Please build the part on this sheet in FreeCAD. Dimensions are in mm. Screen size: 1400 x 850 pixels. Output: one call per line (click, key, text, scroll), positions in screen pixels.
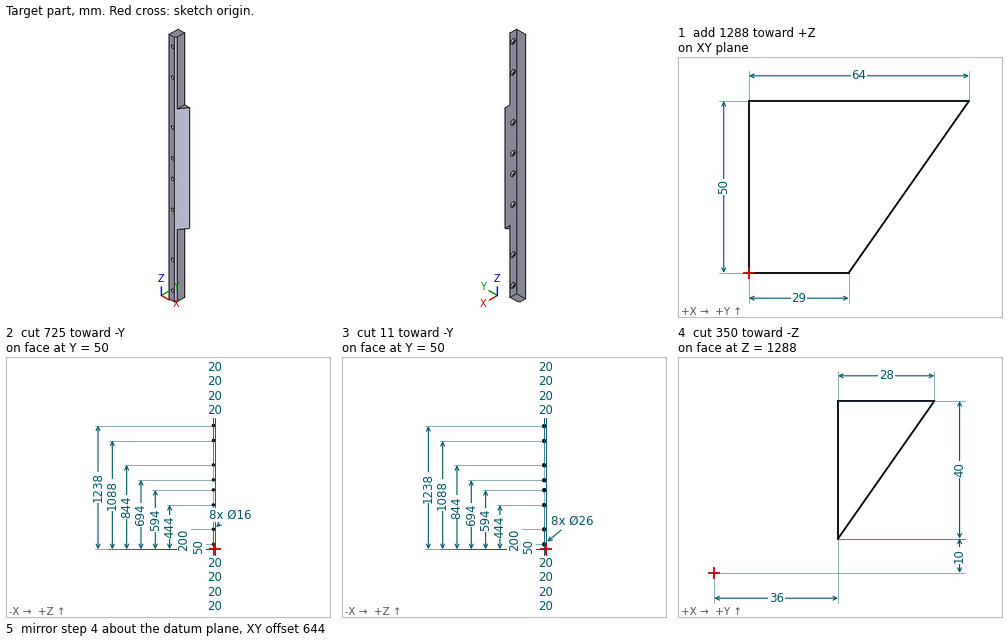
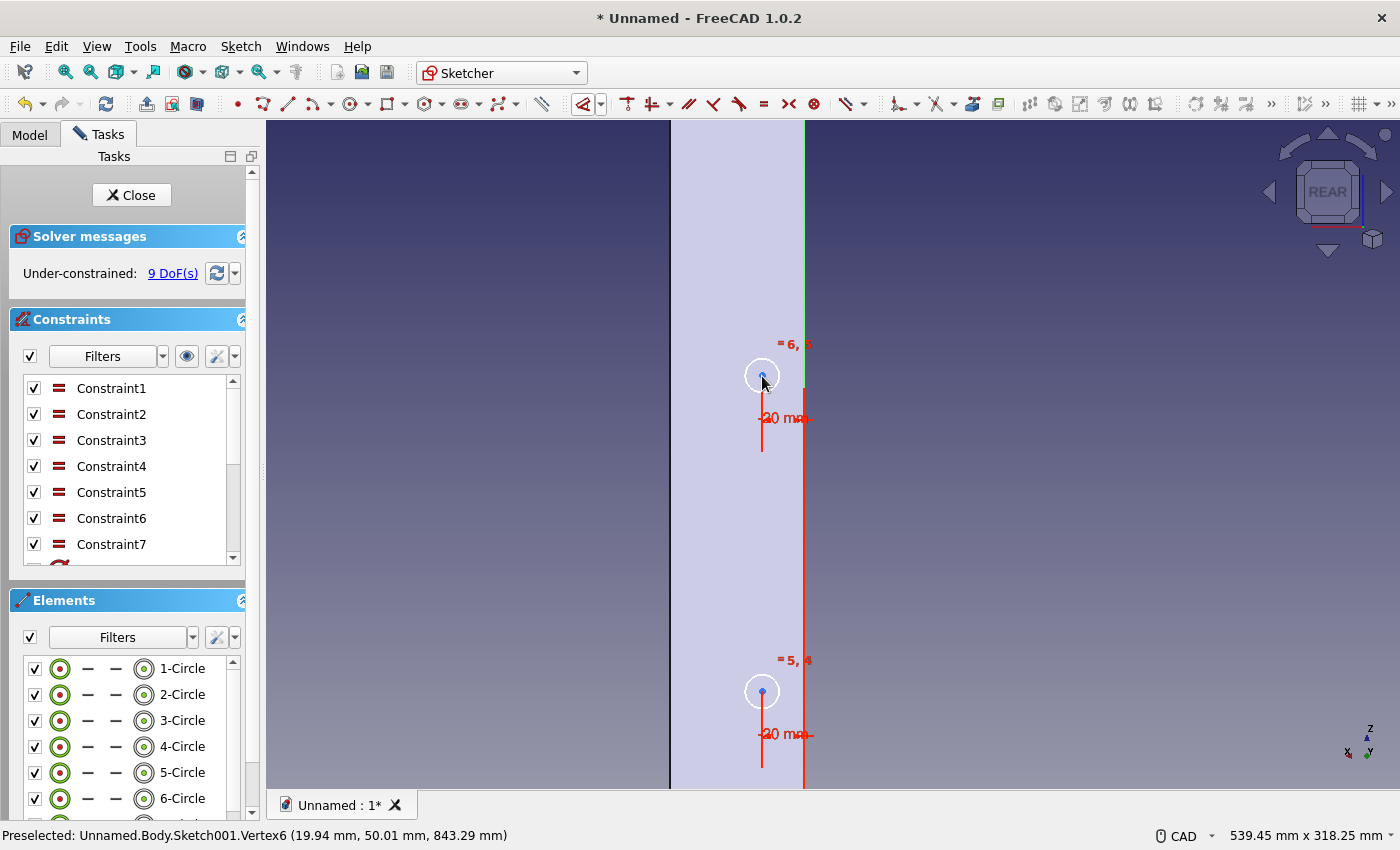
scroll(762, 378, down, 9)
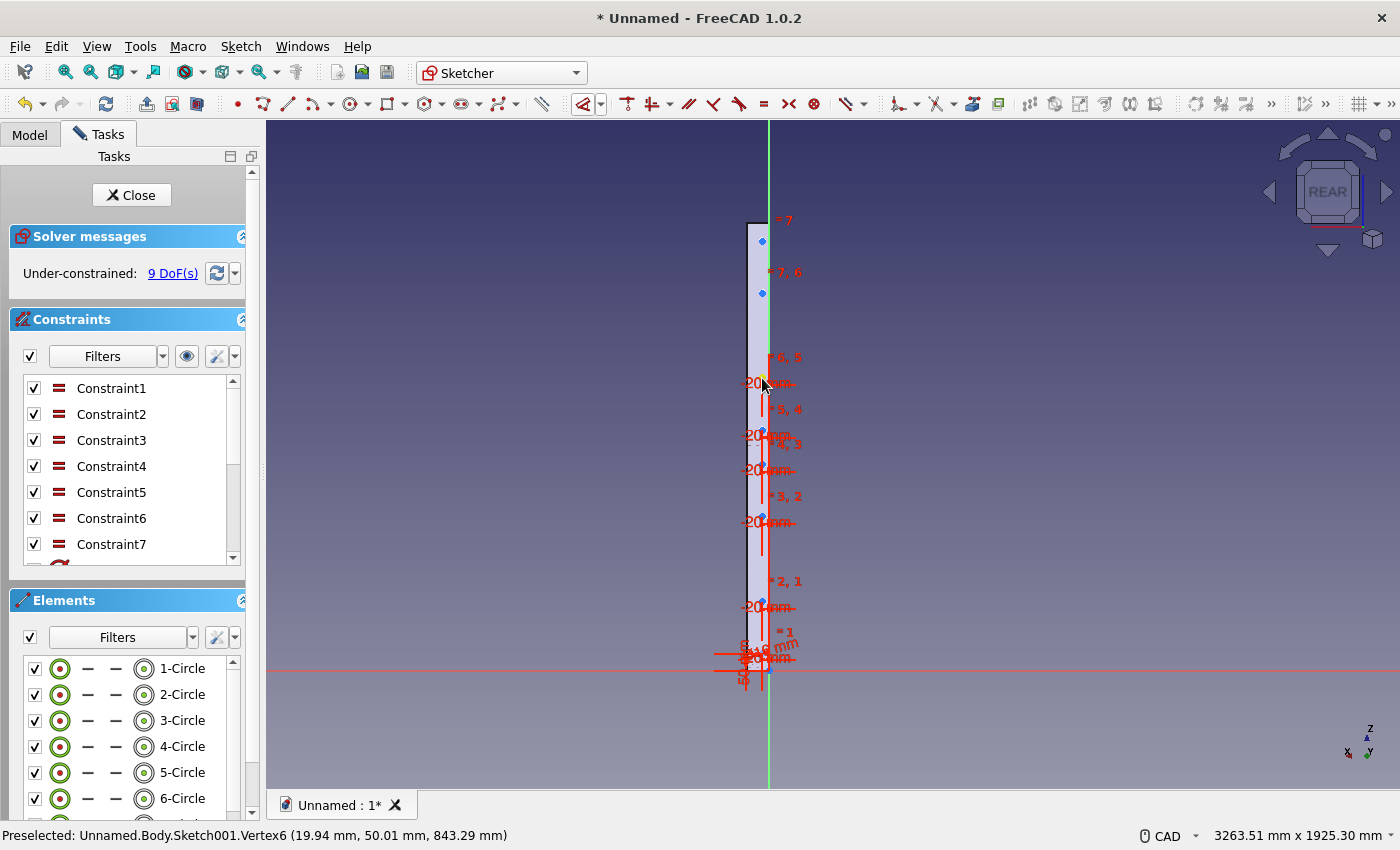
scroll(763, 293, up, 9)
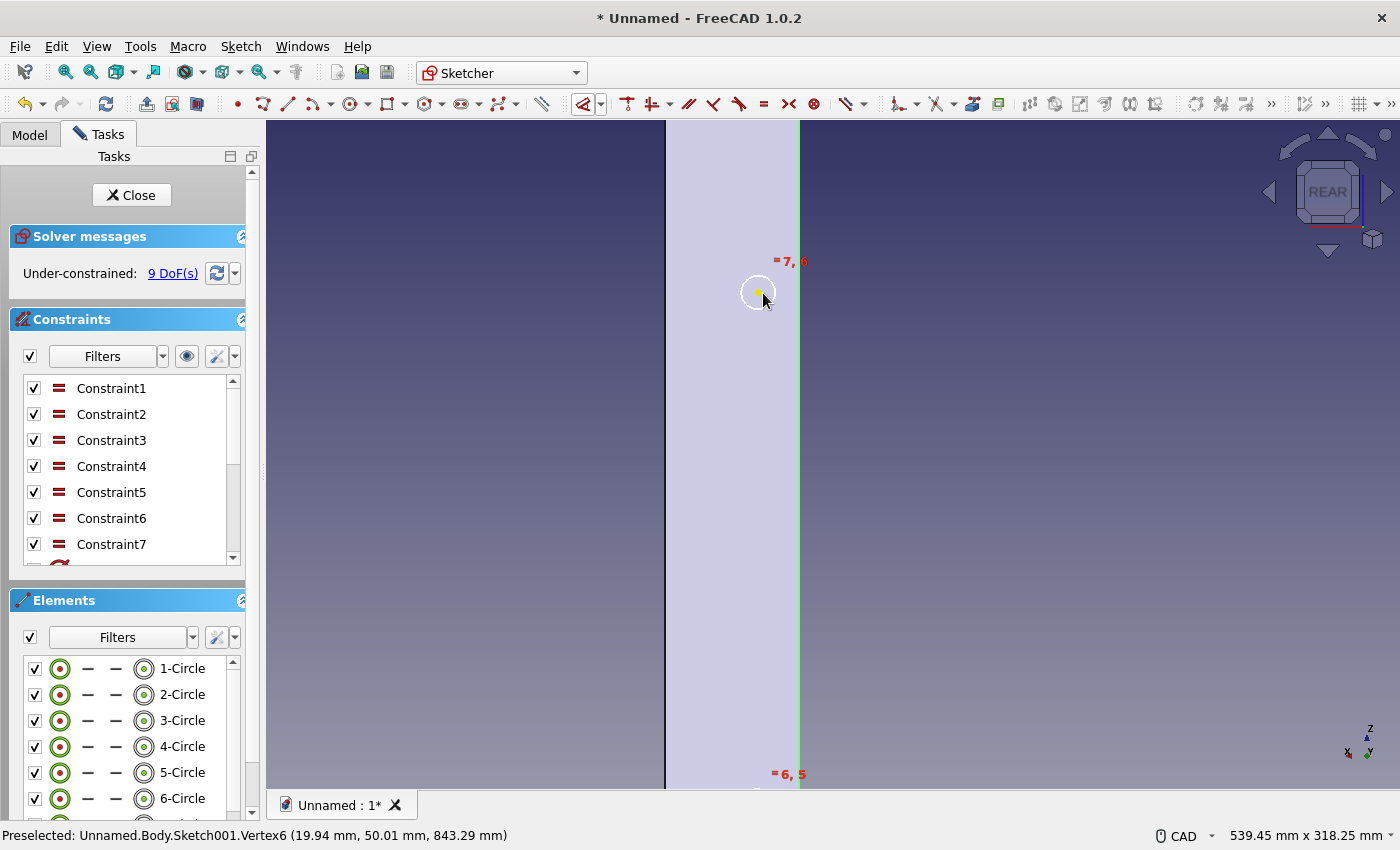
click(758, 293)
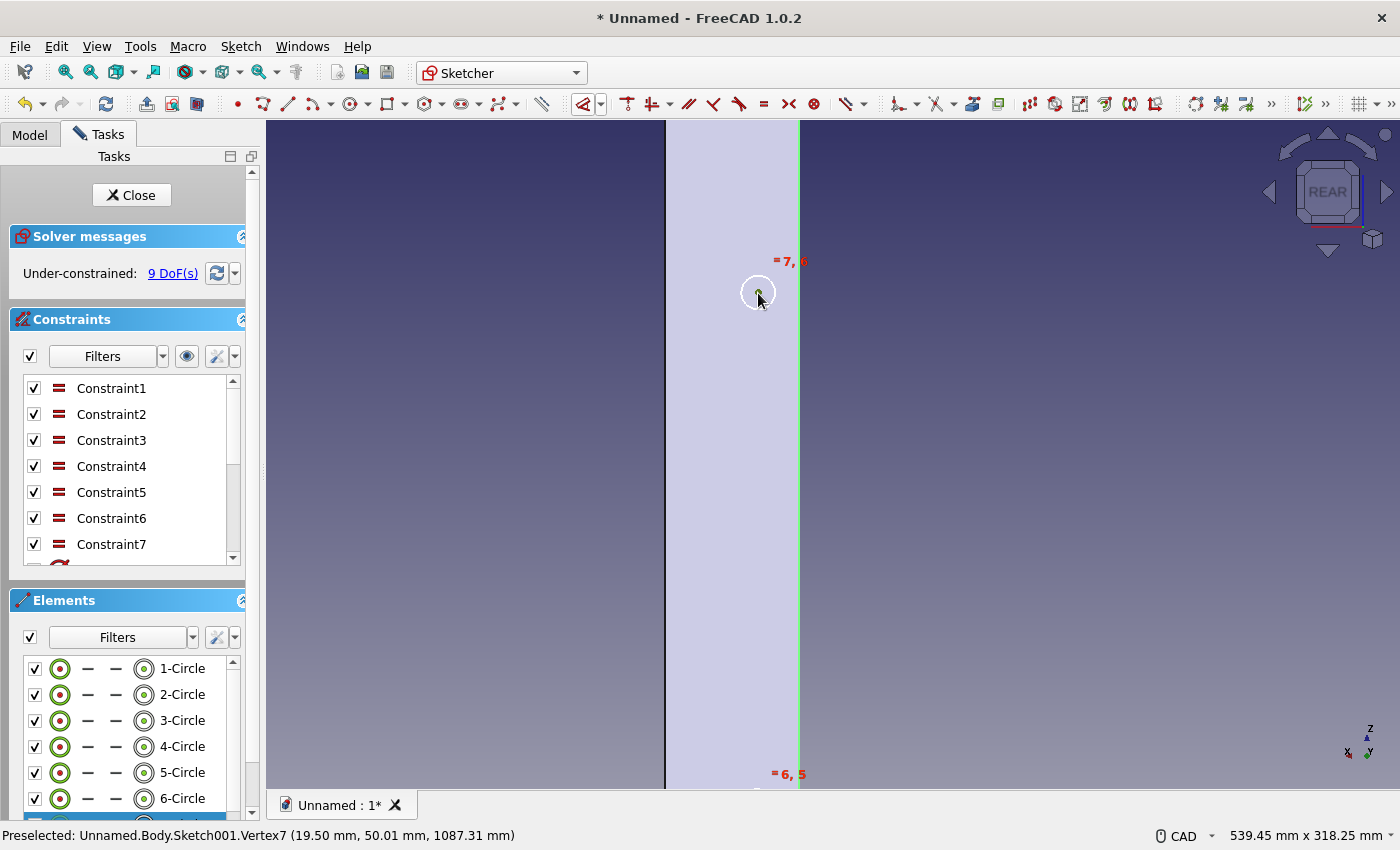
key(l)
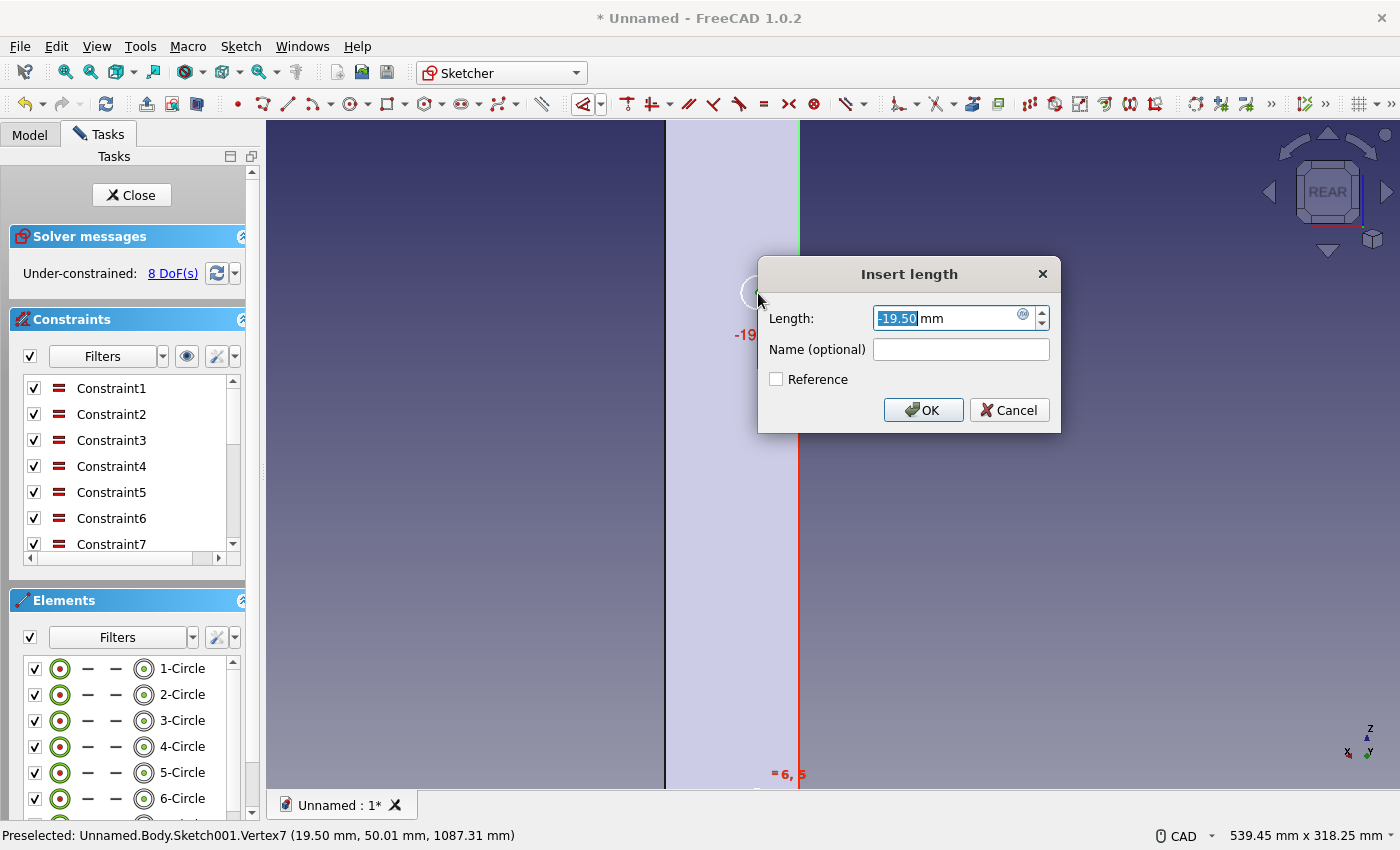
text(-20)
key(Return)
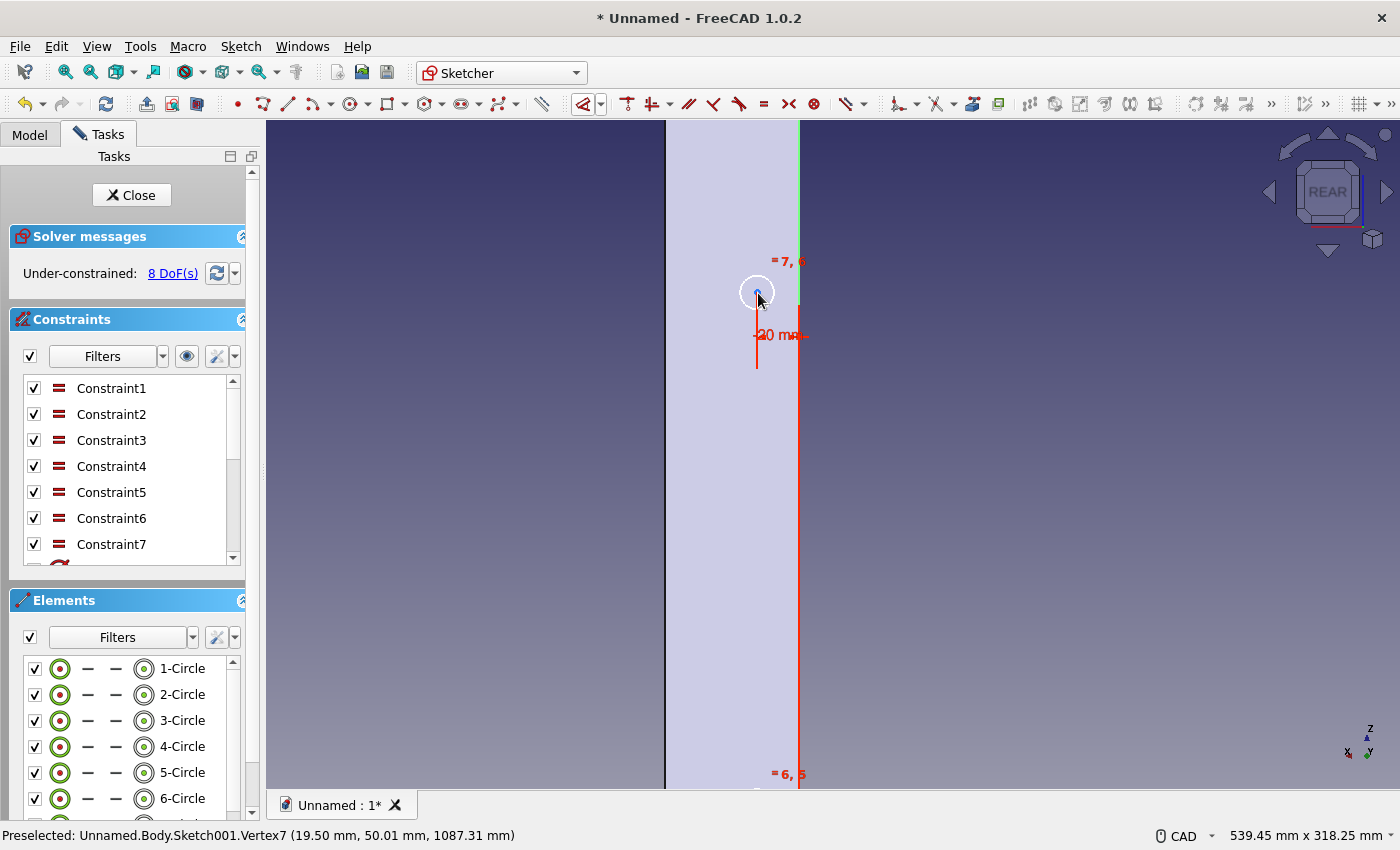
scroll(763, 293, down, 9)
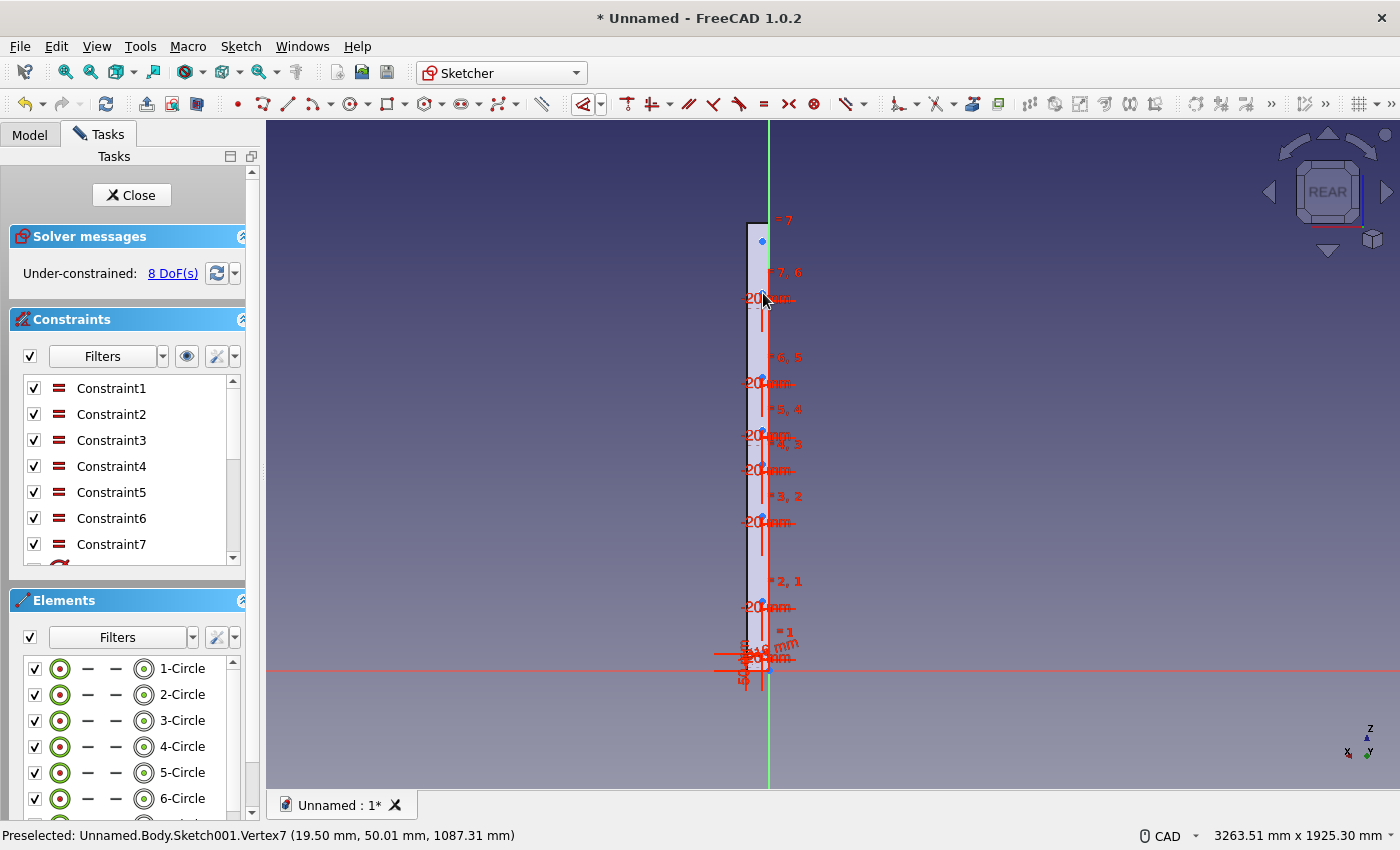
scroll(762, 241, up, 9)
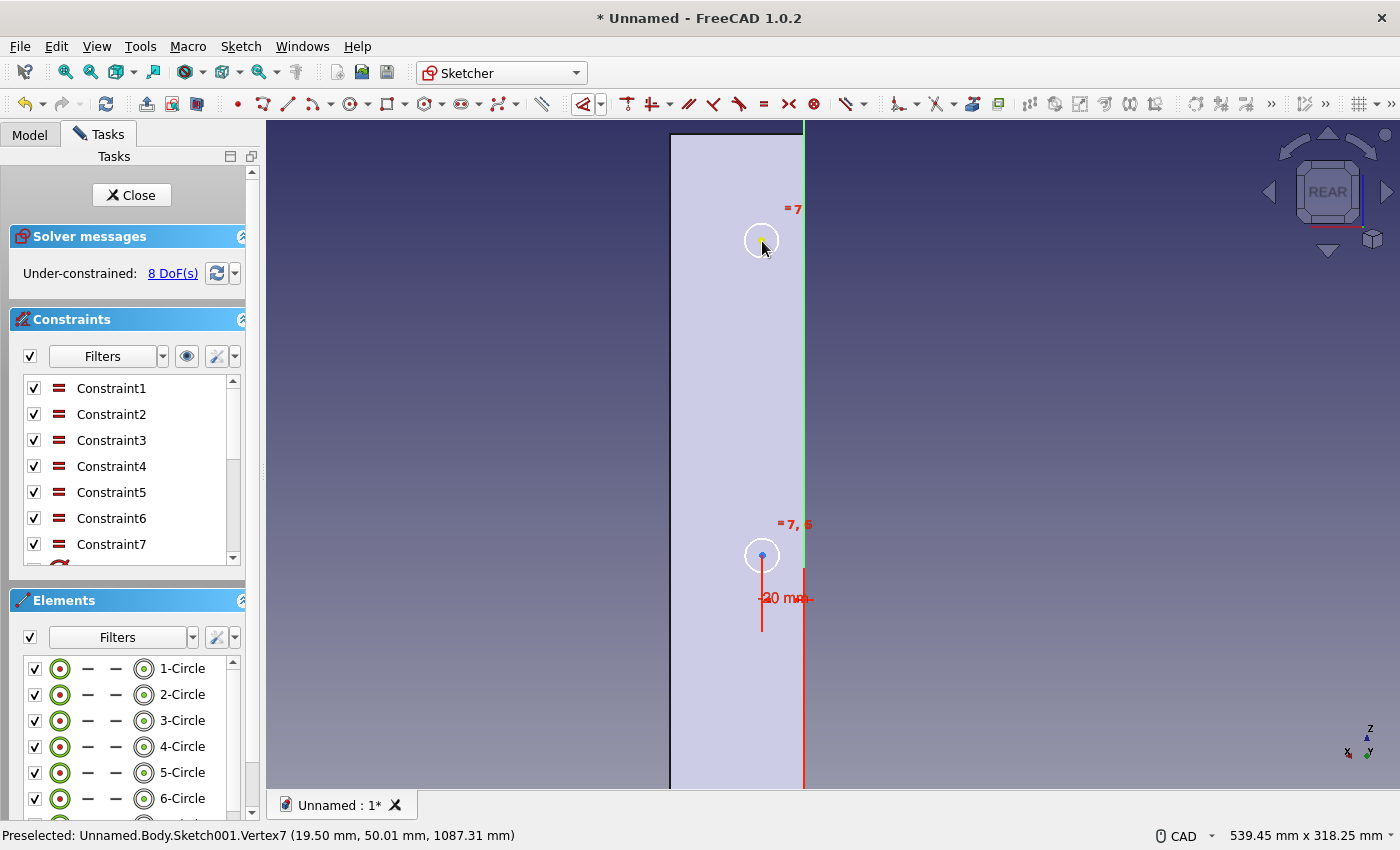
click(762, 241)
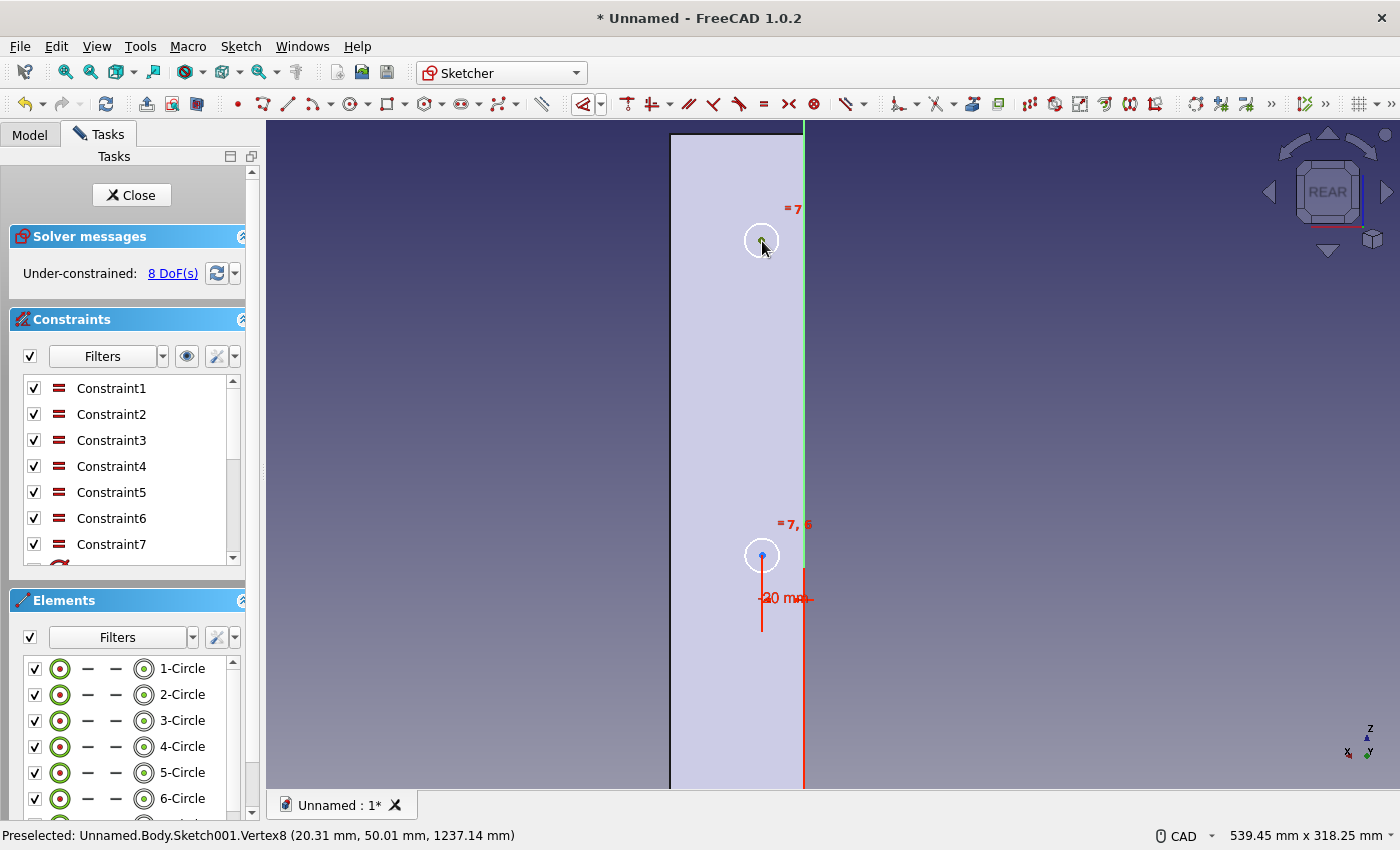
key(l)